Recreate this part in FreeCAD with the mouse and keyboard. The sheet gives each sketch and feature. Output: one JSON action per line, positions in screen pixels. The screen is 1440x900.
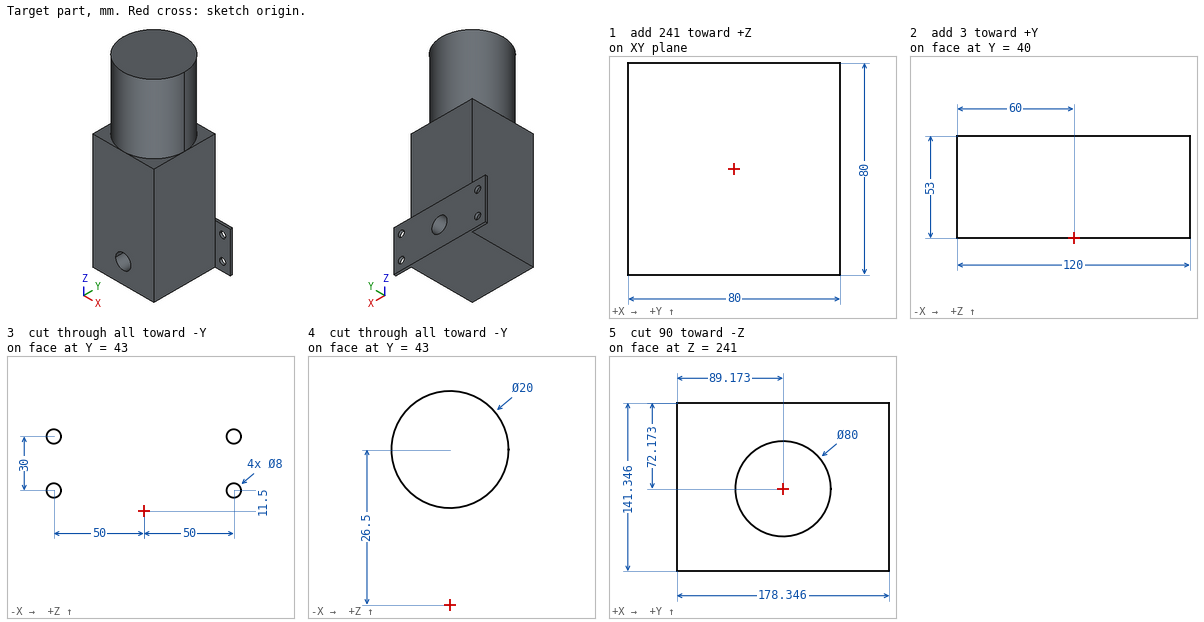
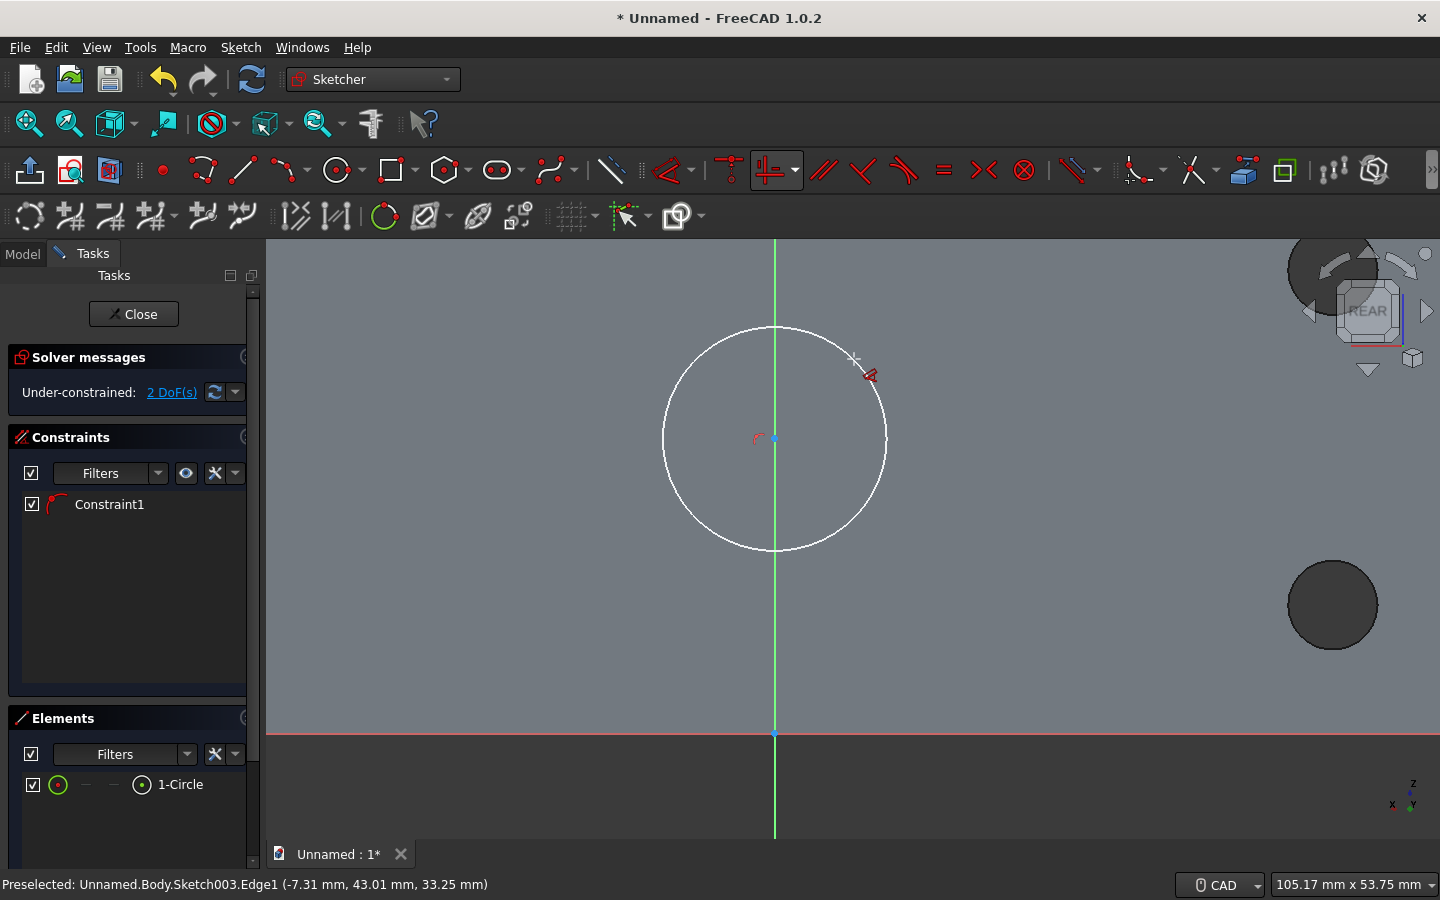
{"action": "left_click", "coordinate": [854, 360]}
{"action": "left_click", "coordinate": [877, 337]}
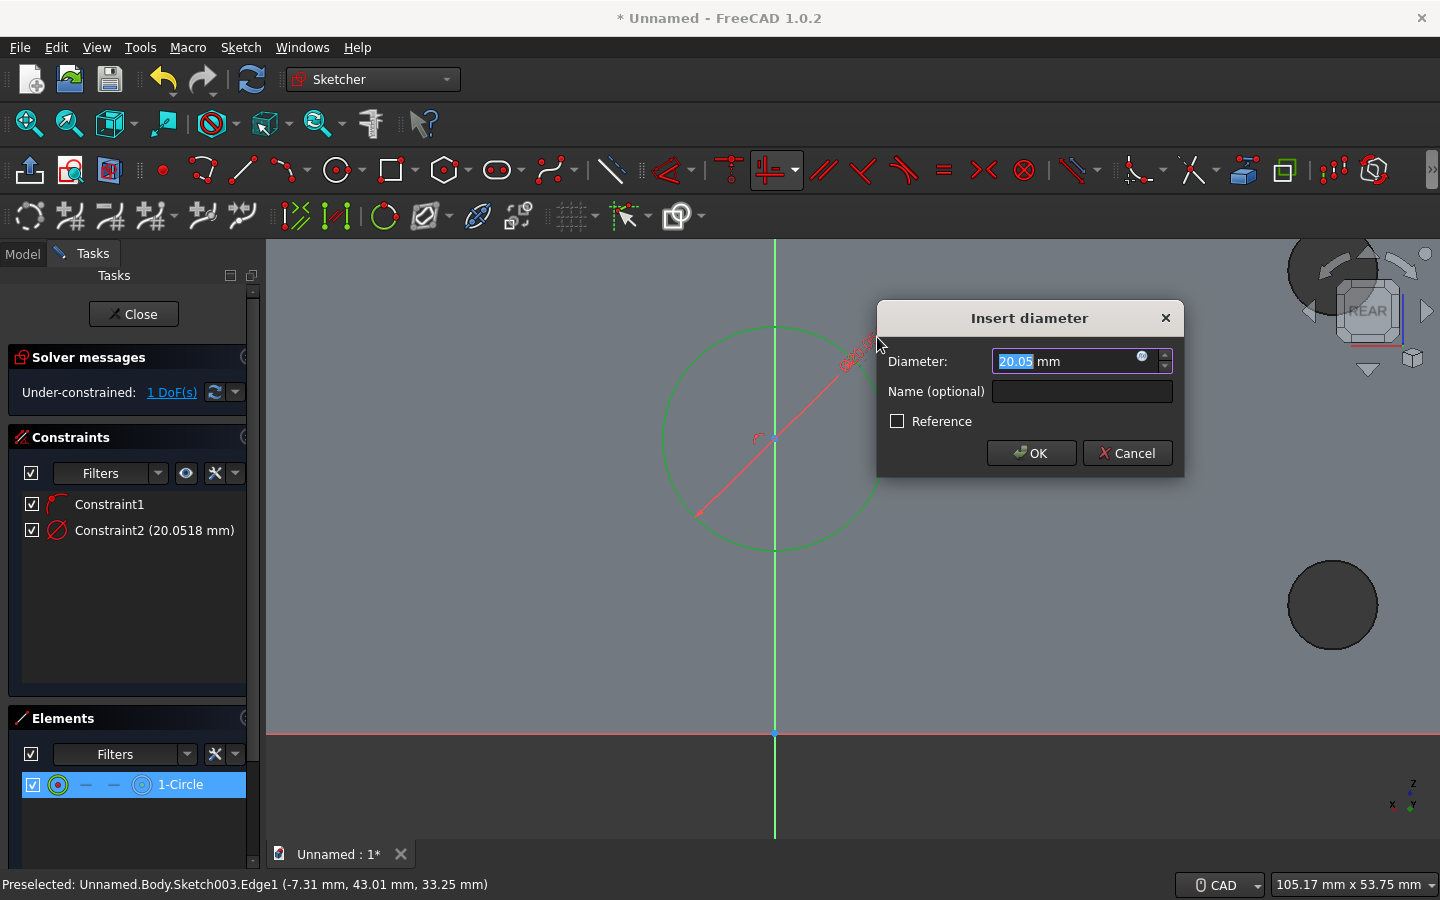
{"action": "type", "text": "20"}
{"action": "key", "text": "Return"}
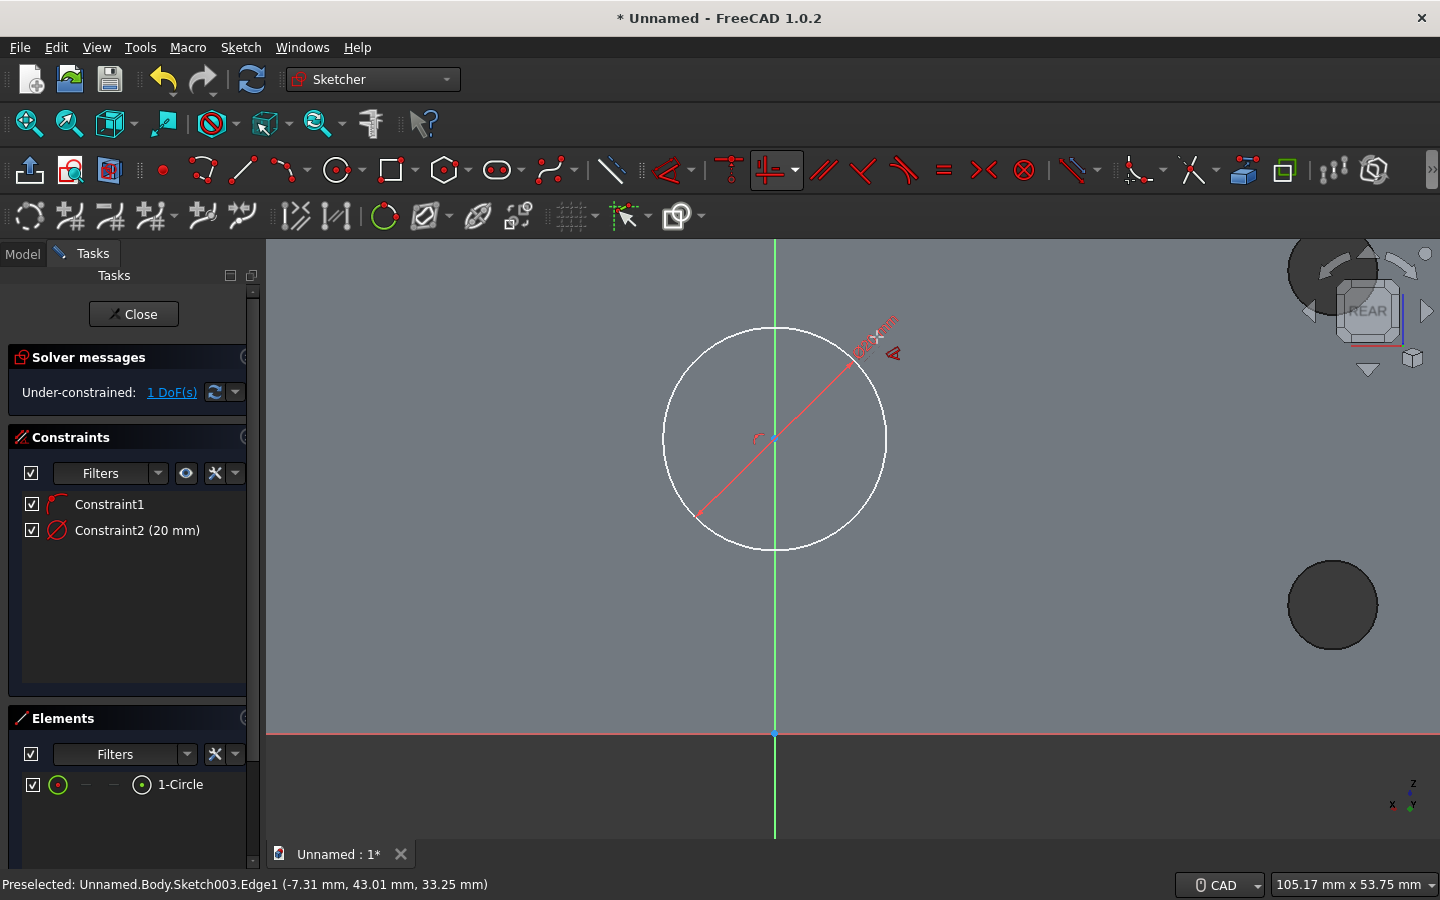
{"action": "left_click", "coordinate": [775, 439]}
{"action": "left_click", "coordinate": [809, 586]}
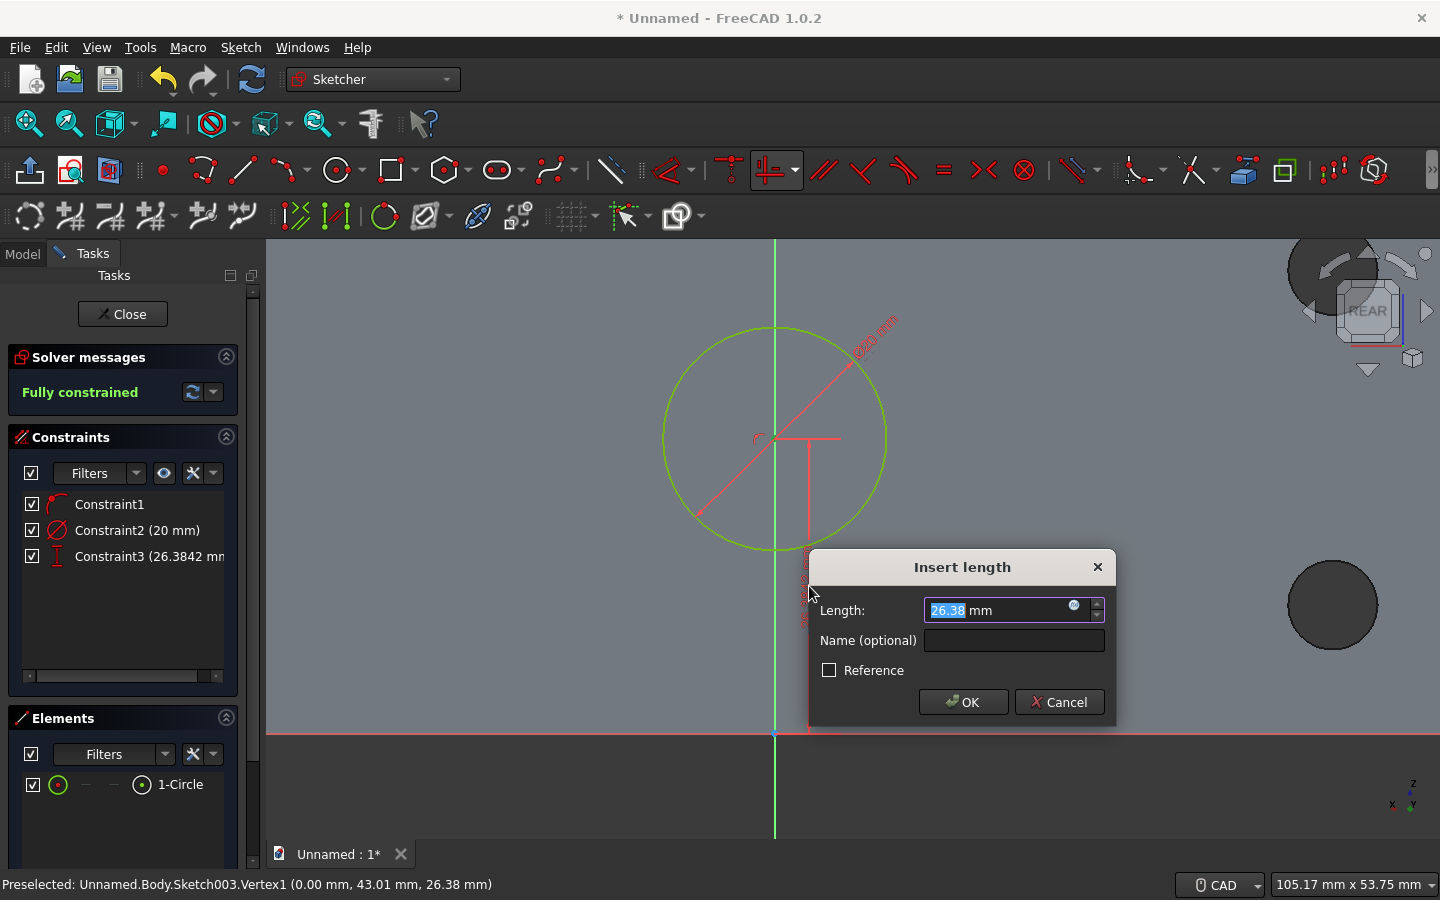
{"action": "type", "text": "26.5"}
{"action": "key", "text": "Return"}
{"action": "key", "text": "Escape"}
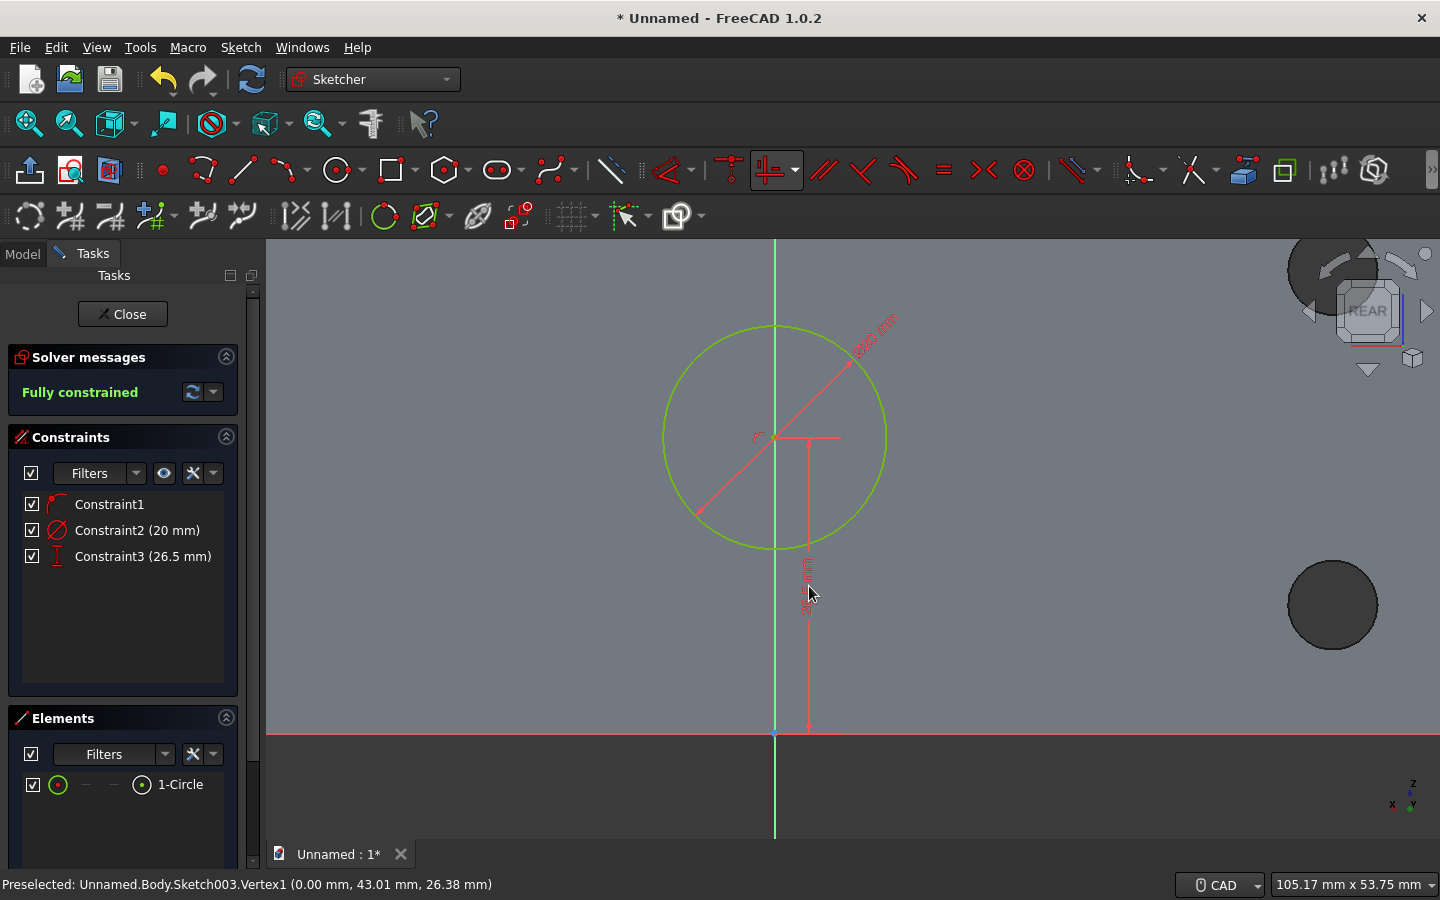
{"action": "left_click", "coordinate": [123, 314]}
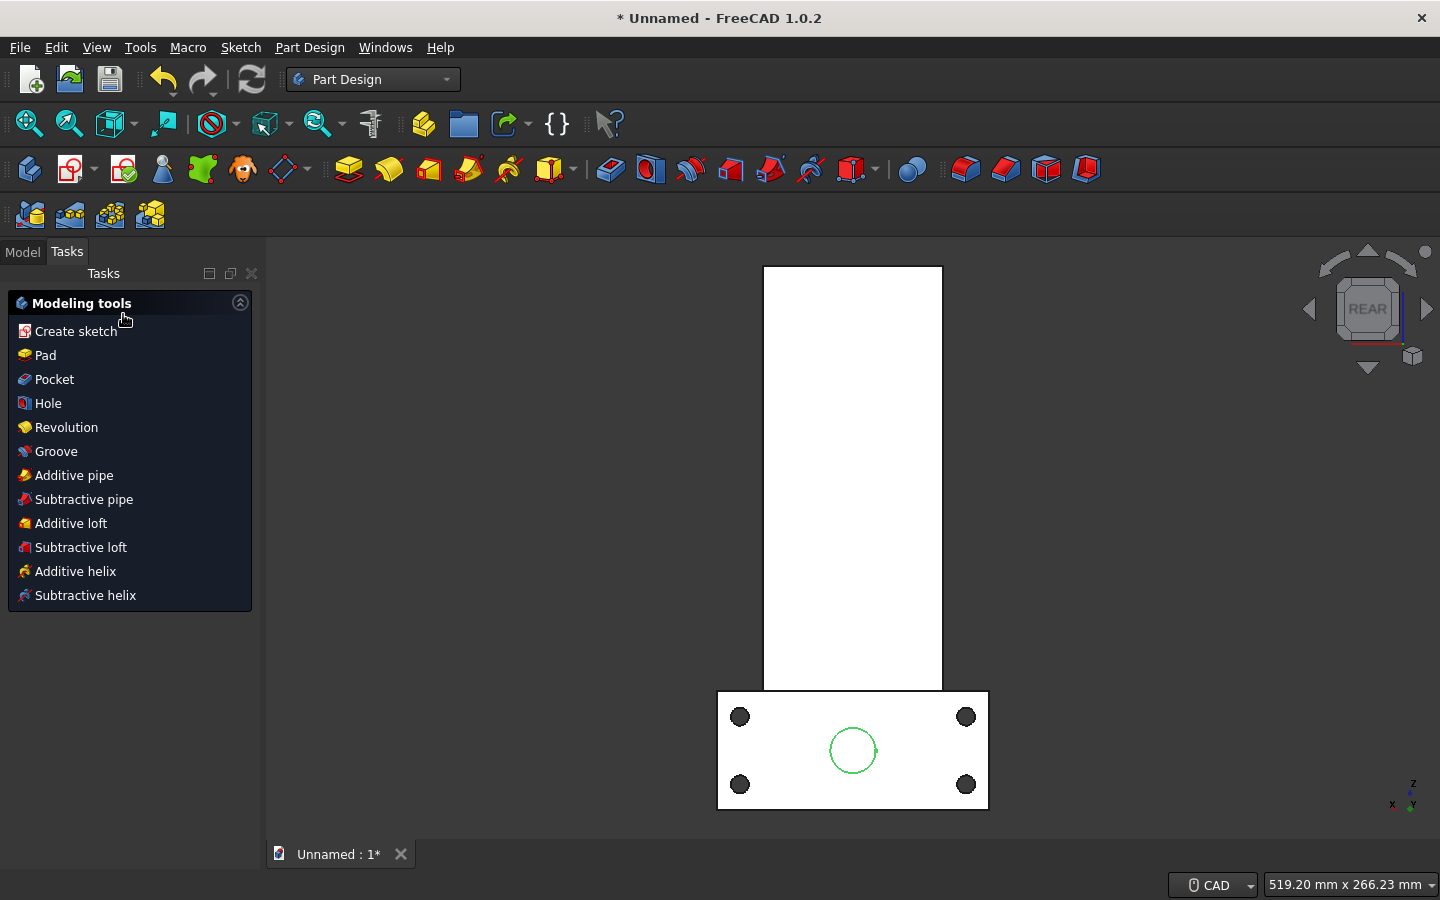
{"action": "left_click", "coordinate": [612, 170]}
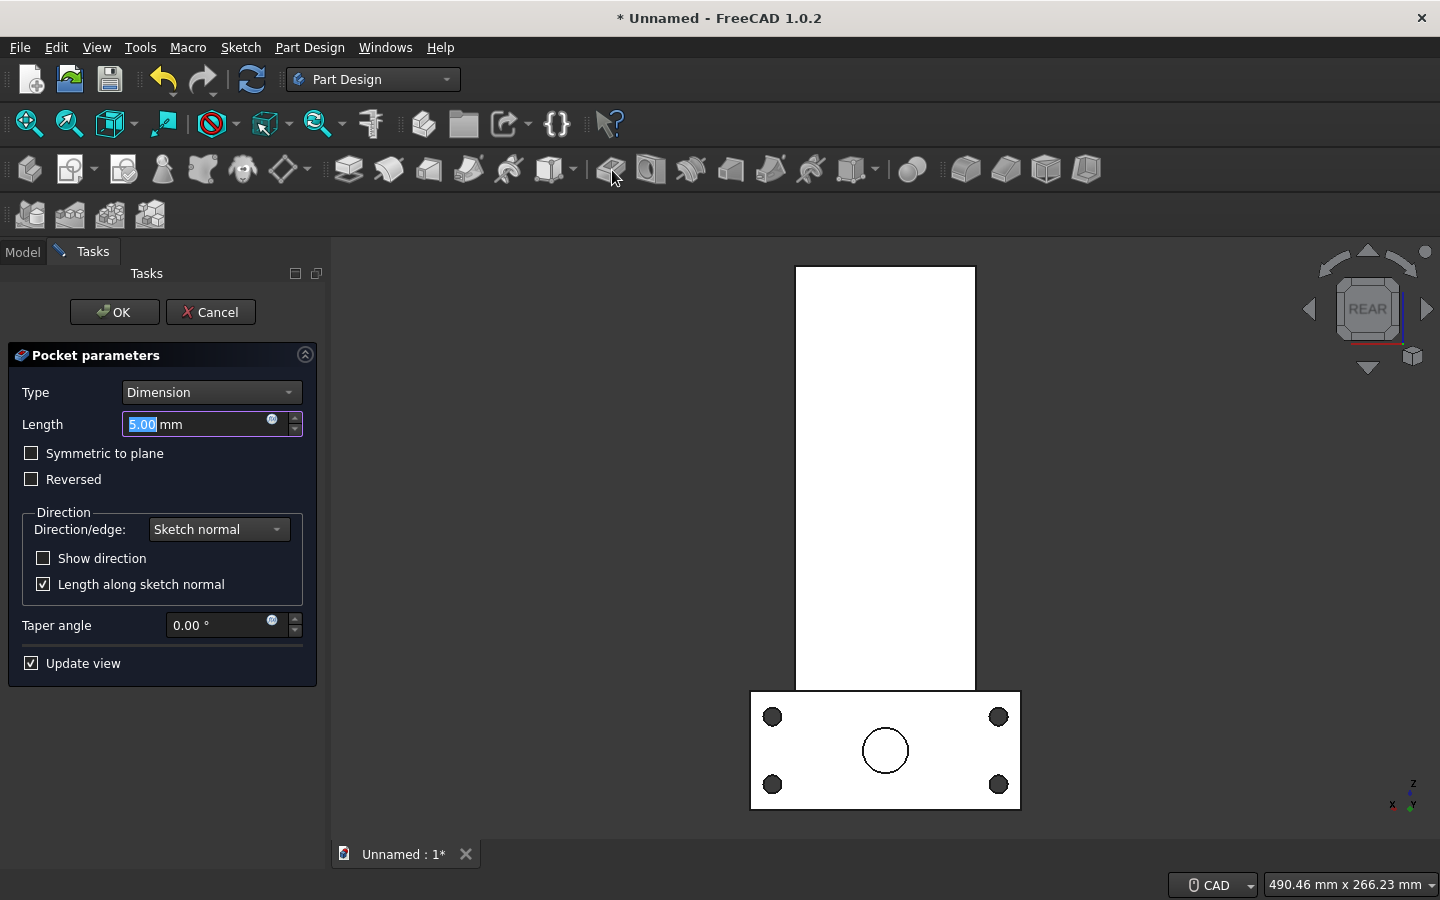
{"action": "left_click", "coordinate": [212, 392]}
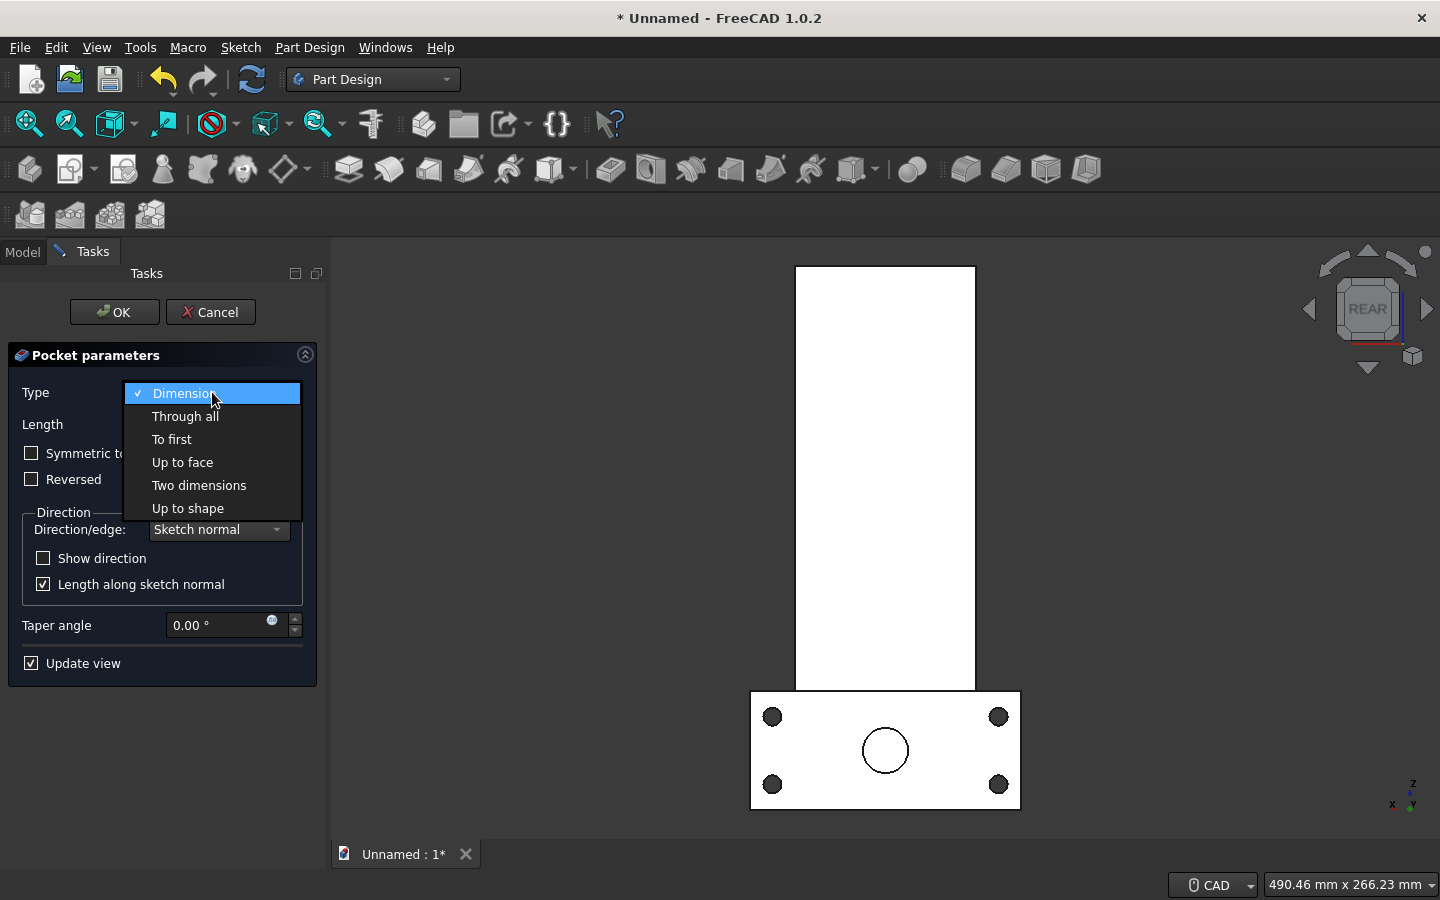
{"action": "left_click", "coordinate": [212, 416]}